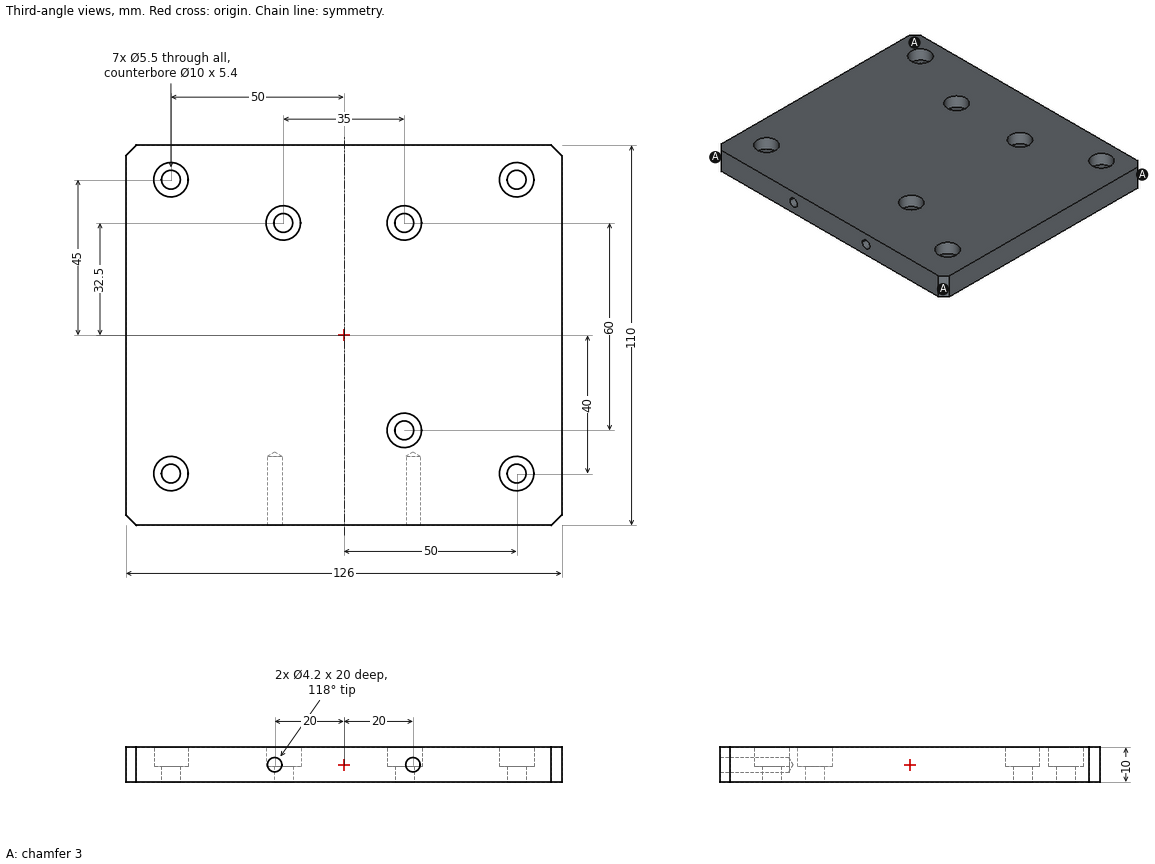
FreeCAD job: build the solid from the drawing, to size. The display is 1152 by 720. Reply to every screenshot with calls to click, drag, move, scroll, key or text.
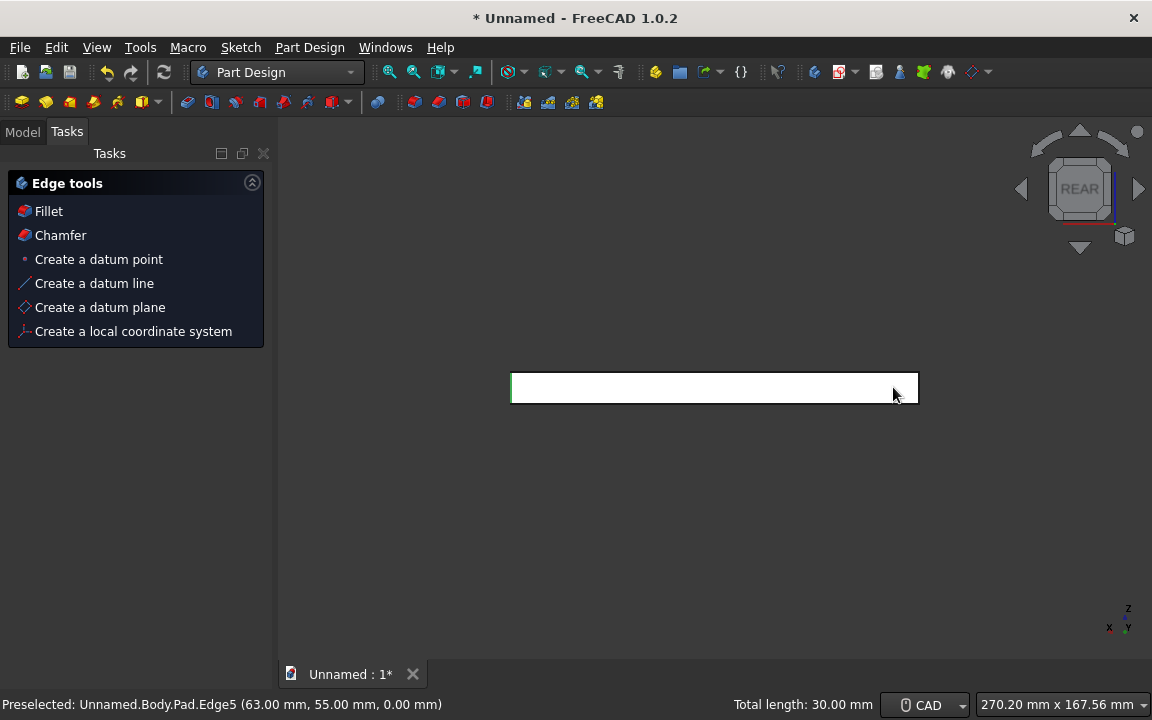
click(919, 387, ctrl)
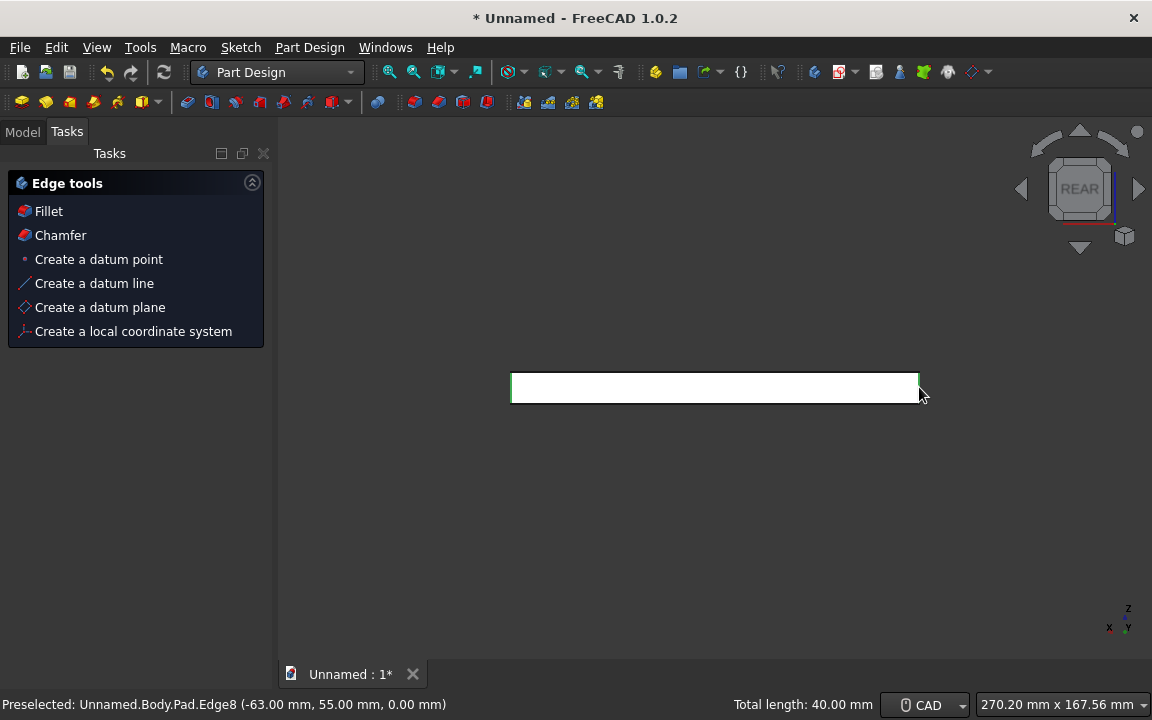
click(440, 102)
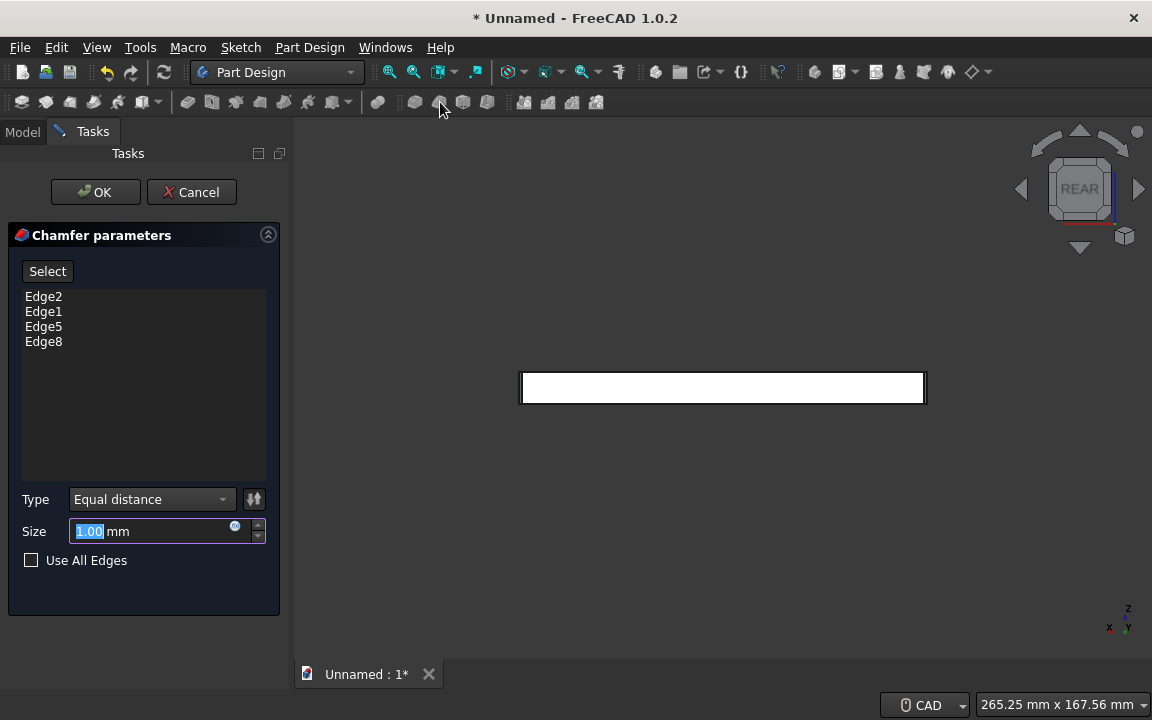
text(3)
key(Tab)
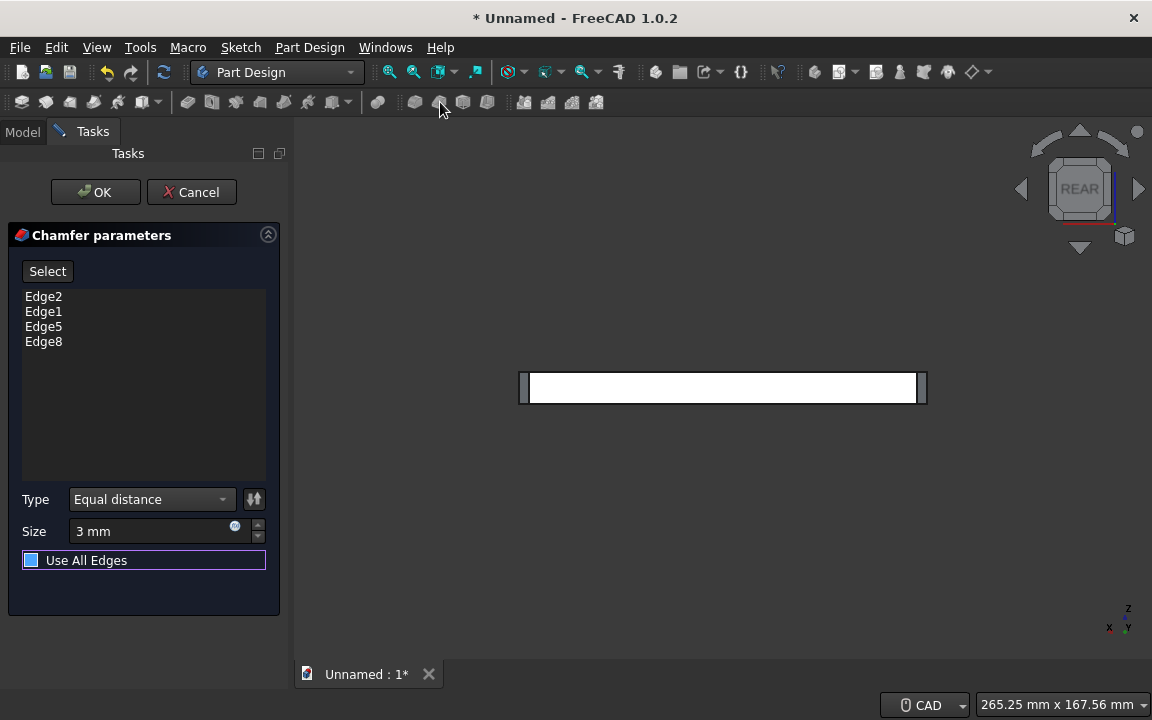
click(96, 192)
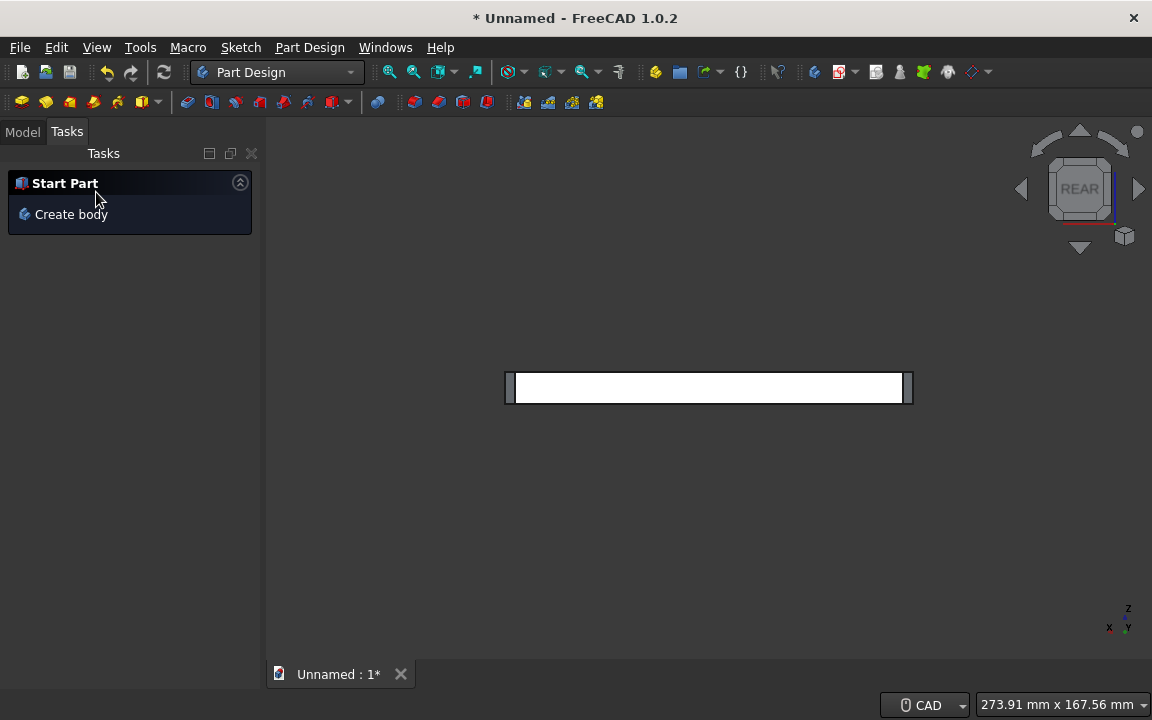
key(0)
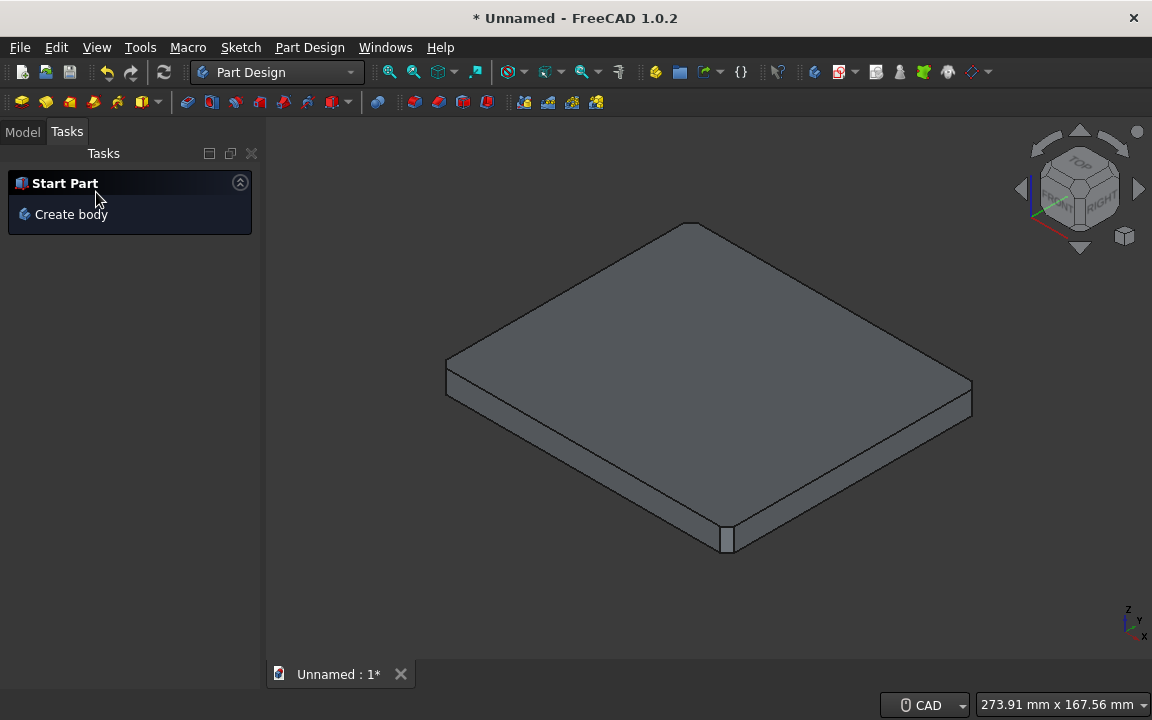
click(709, 374)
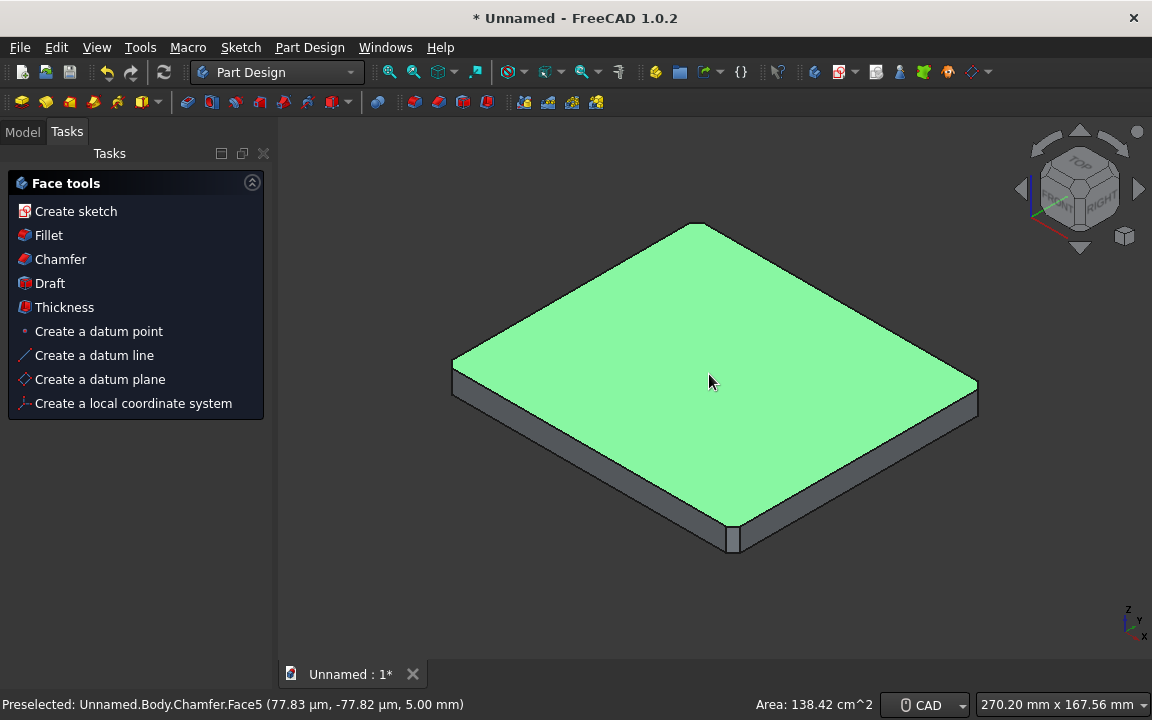
click(840, 72)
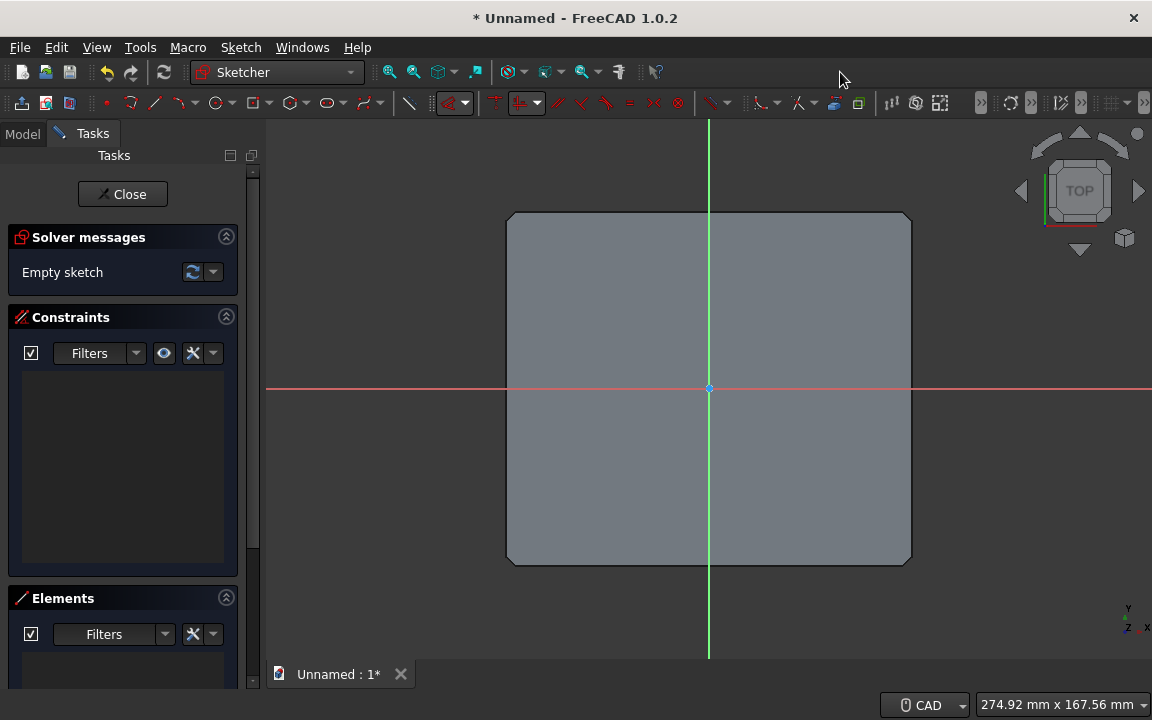
click(216, 104)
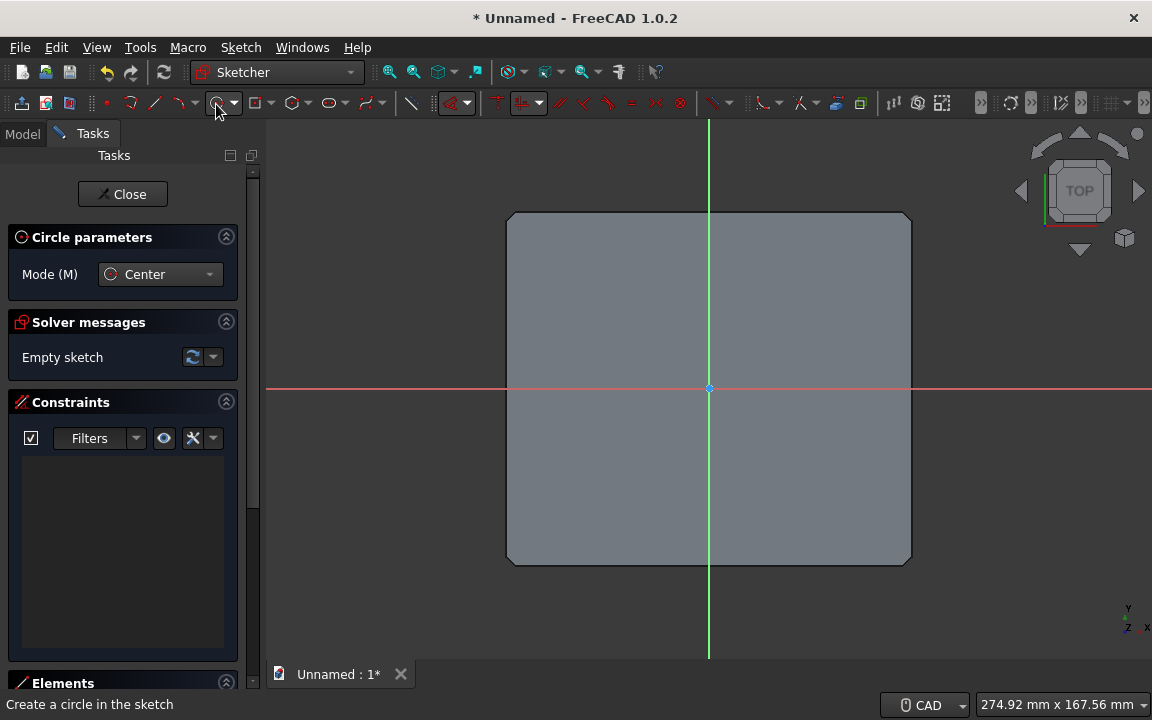
scroll(548, 244, up, 5)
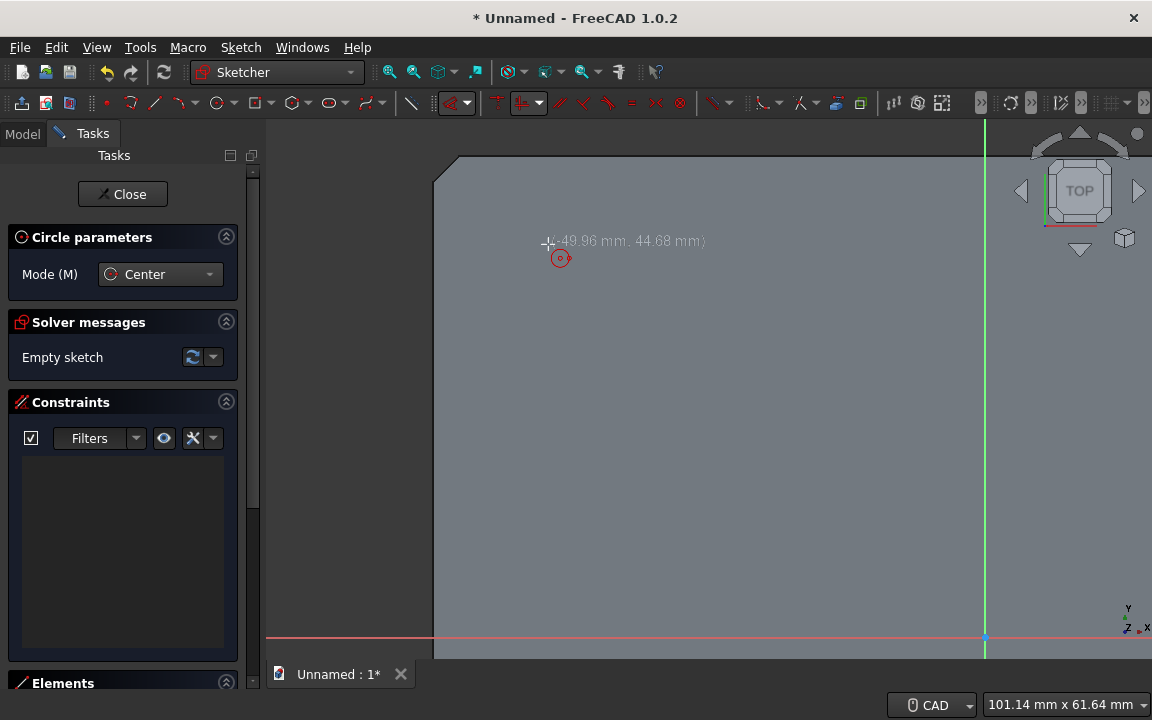
click(547, 244)
move(564, 227)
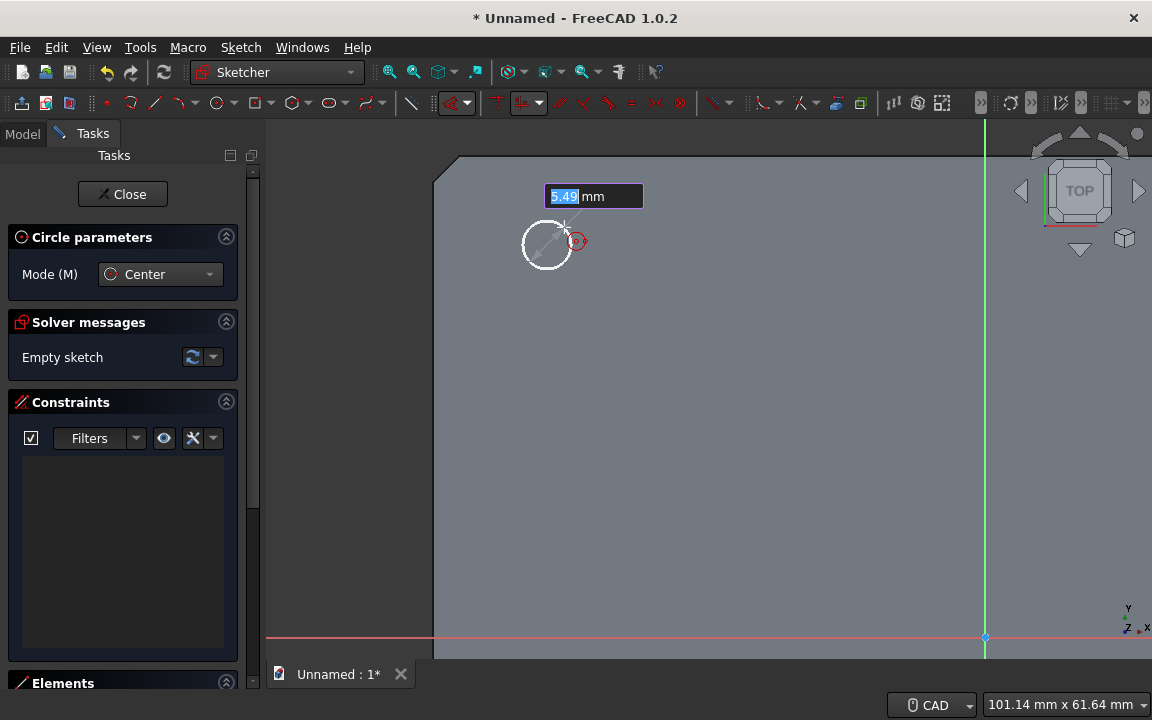
text(5.5)
key(Return)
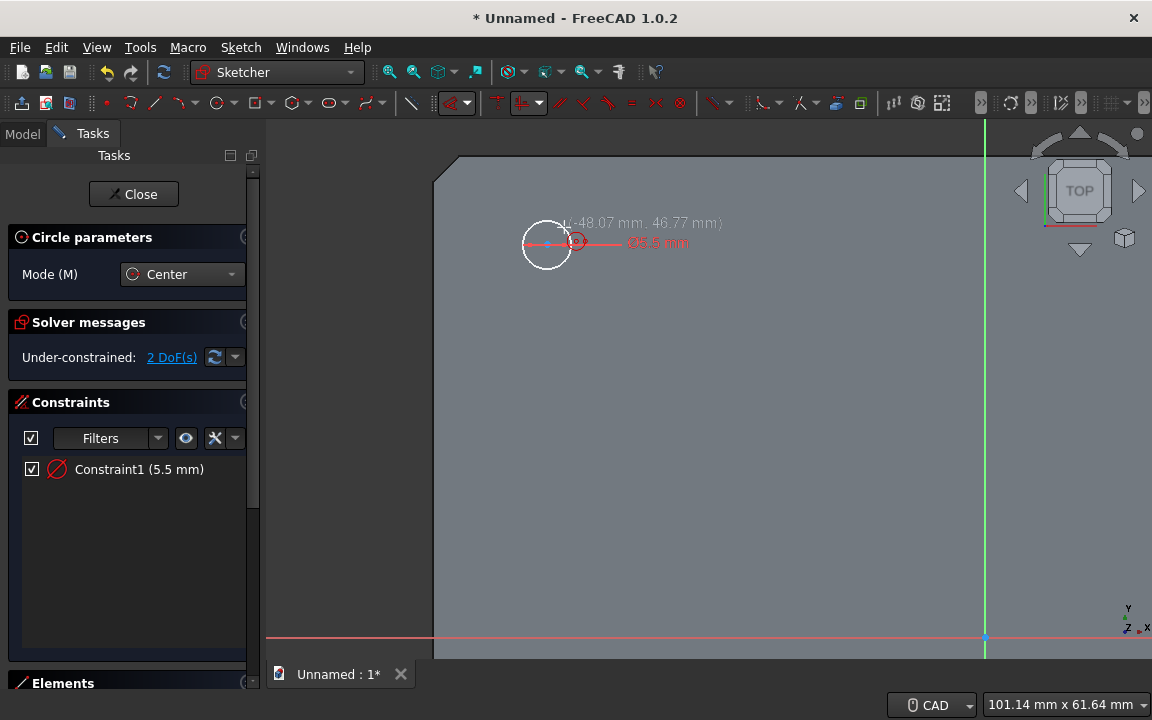
click(832, 353)
move(849, 336)